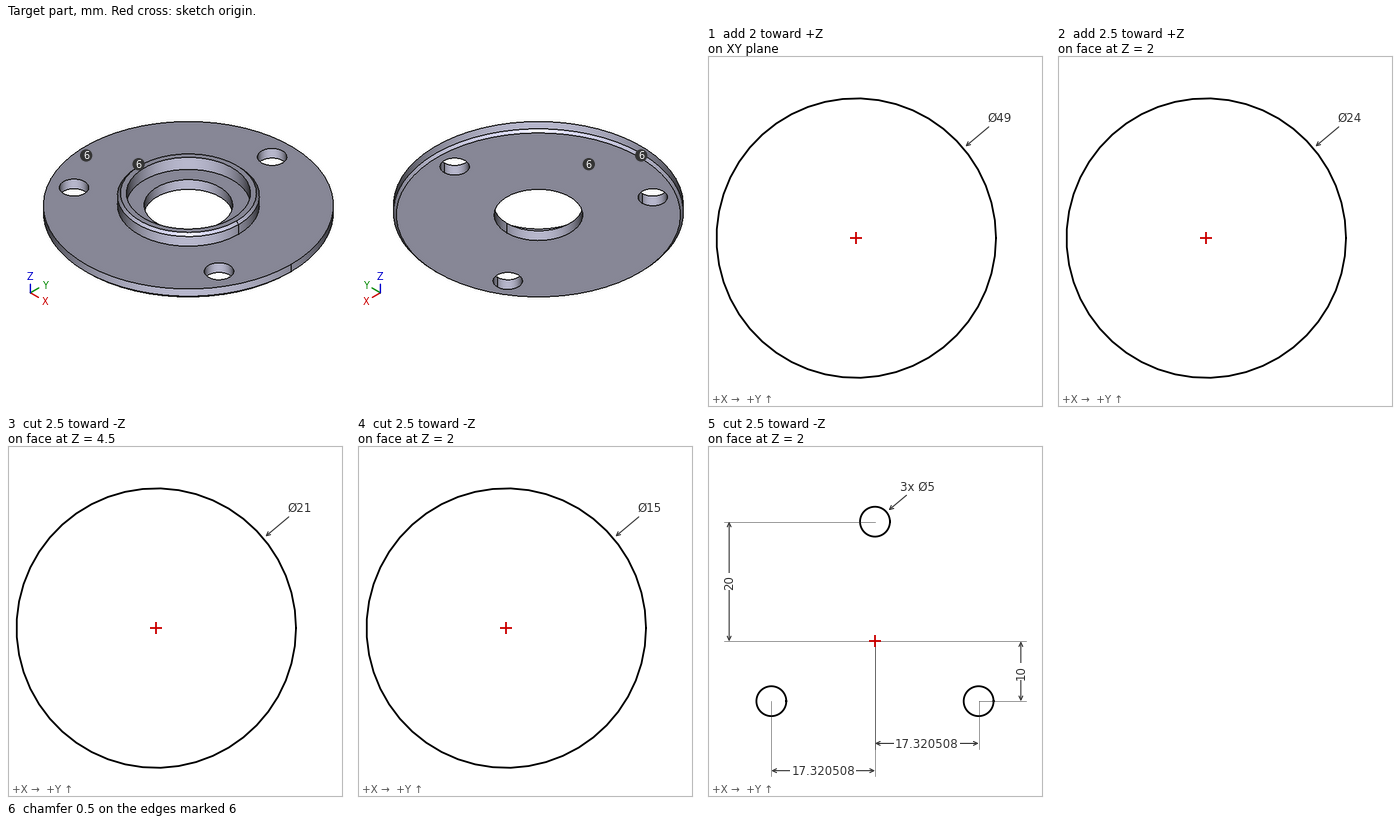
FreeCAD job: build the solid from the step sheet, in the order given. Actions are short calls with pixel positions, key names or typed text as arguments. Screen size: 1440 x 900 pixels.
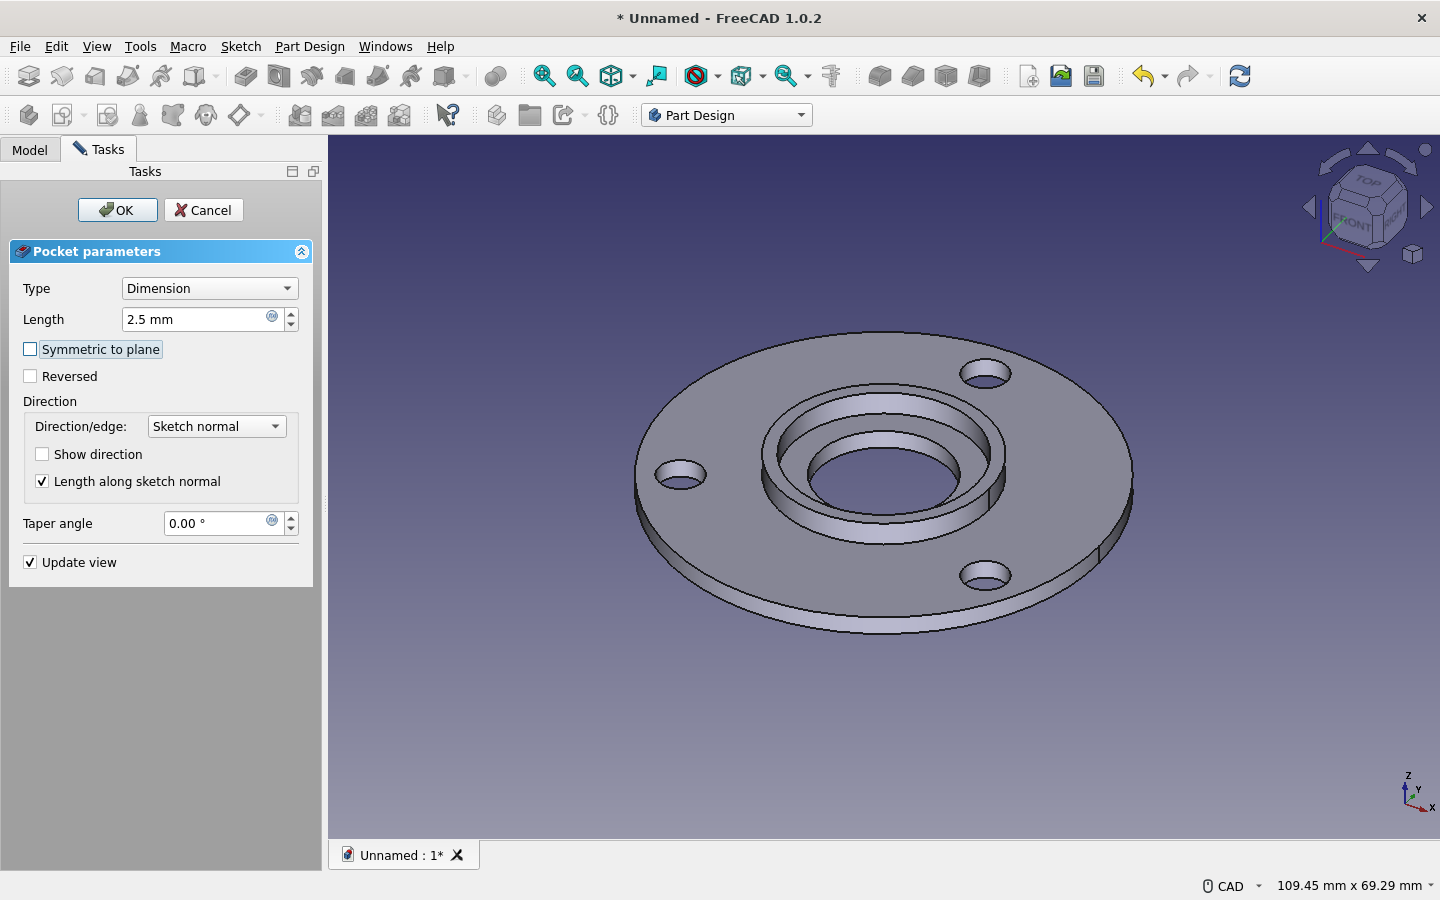
click(118, 210)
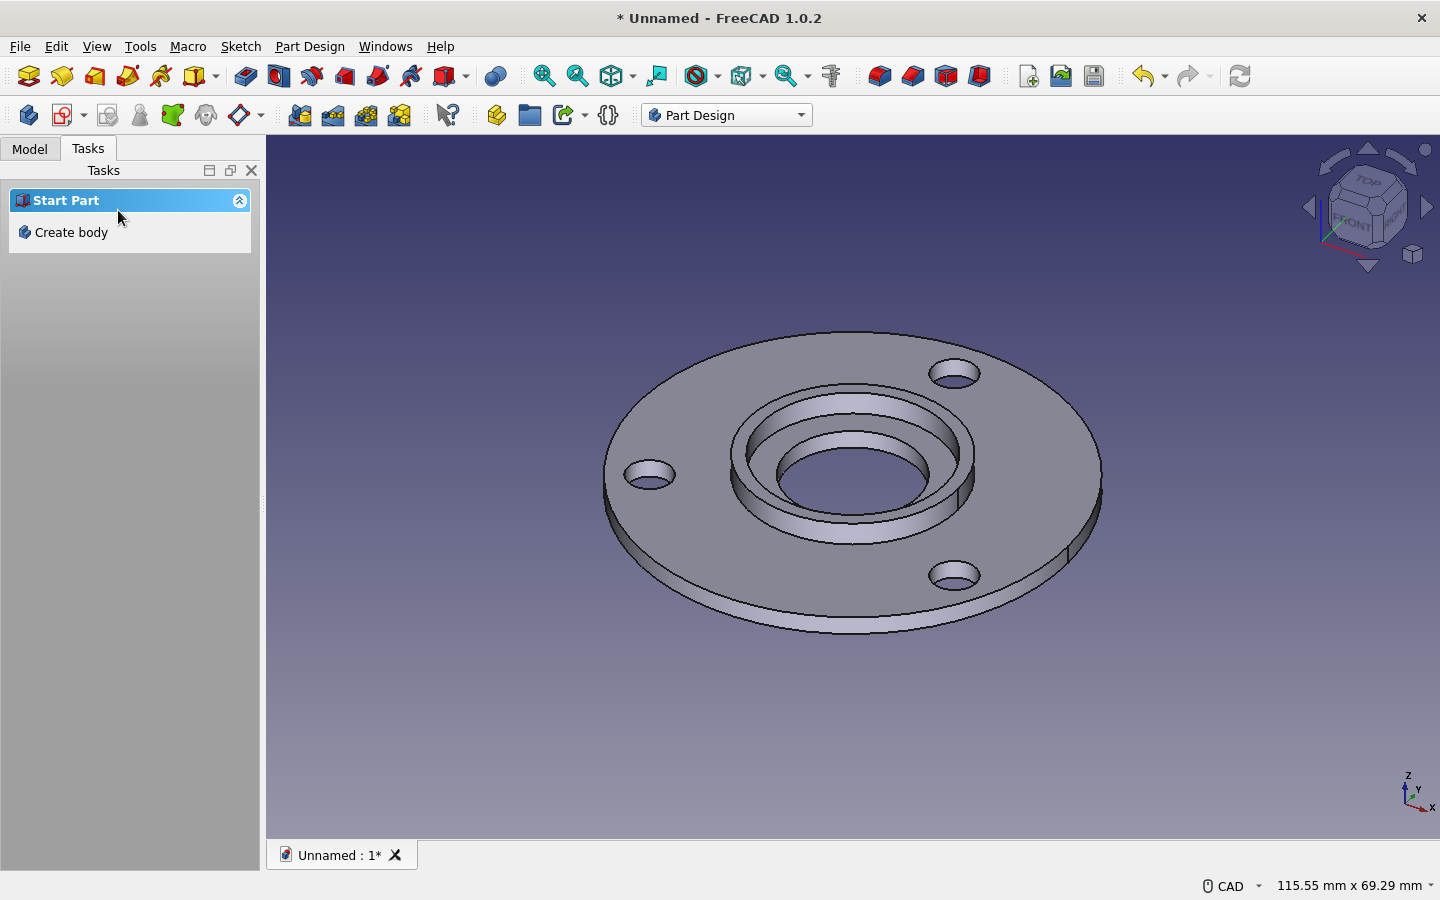
click(732, 460)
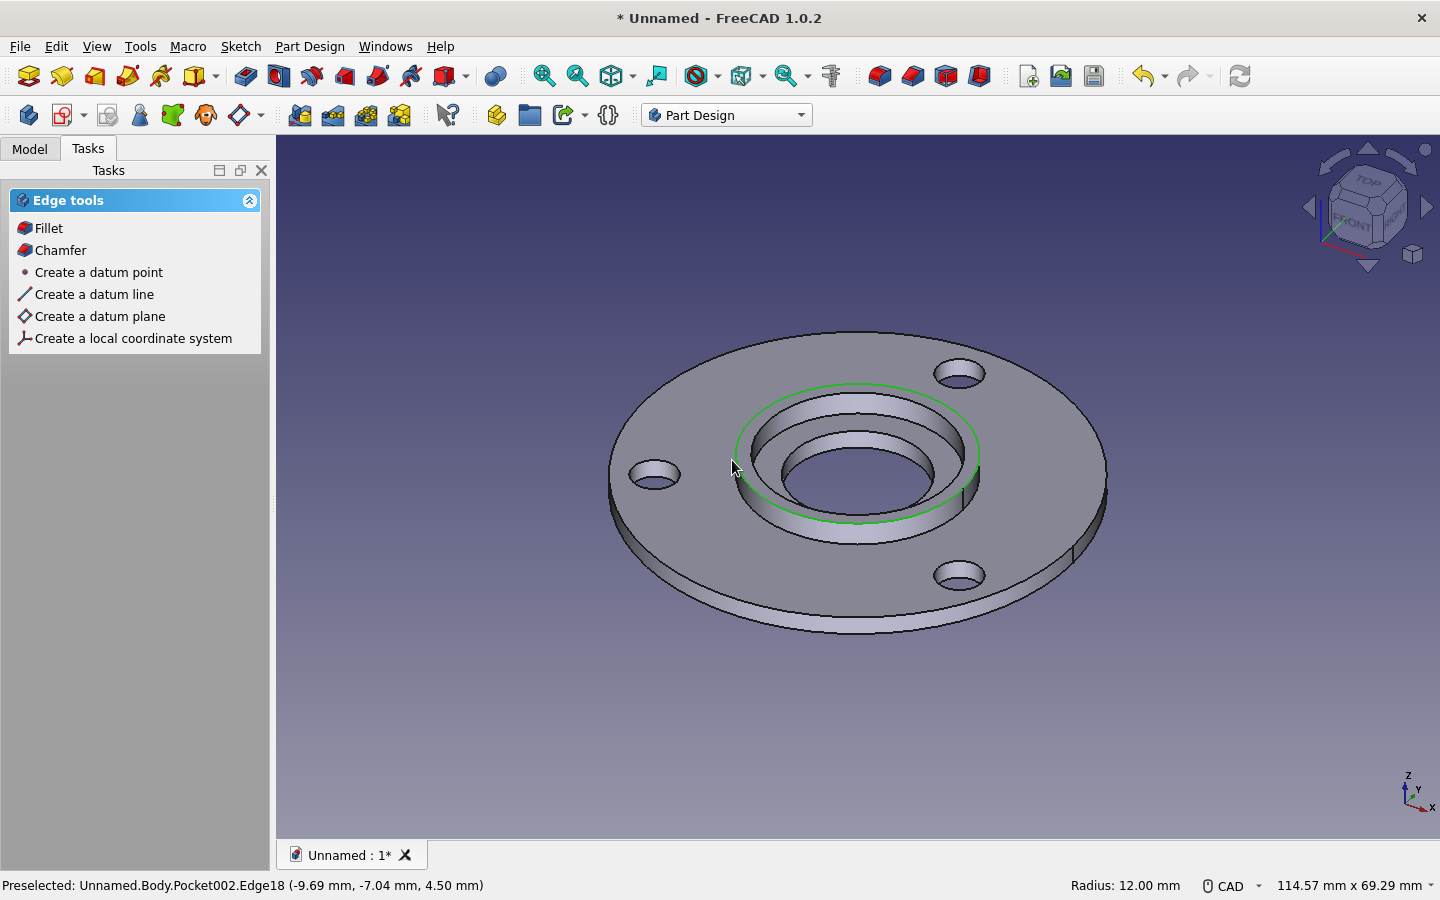
key(0)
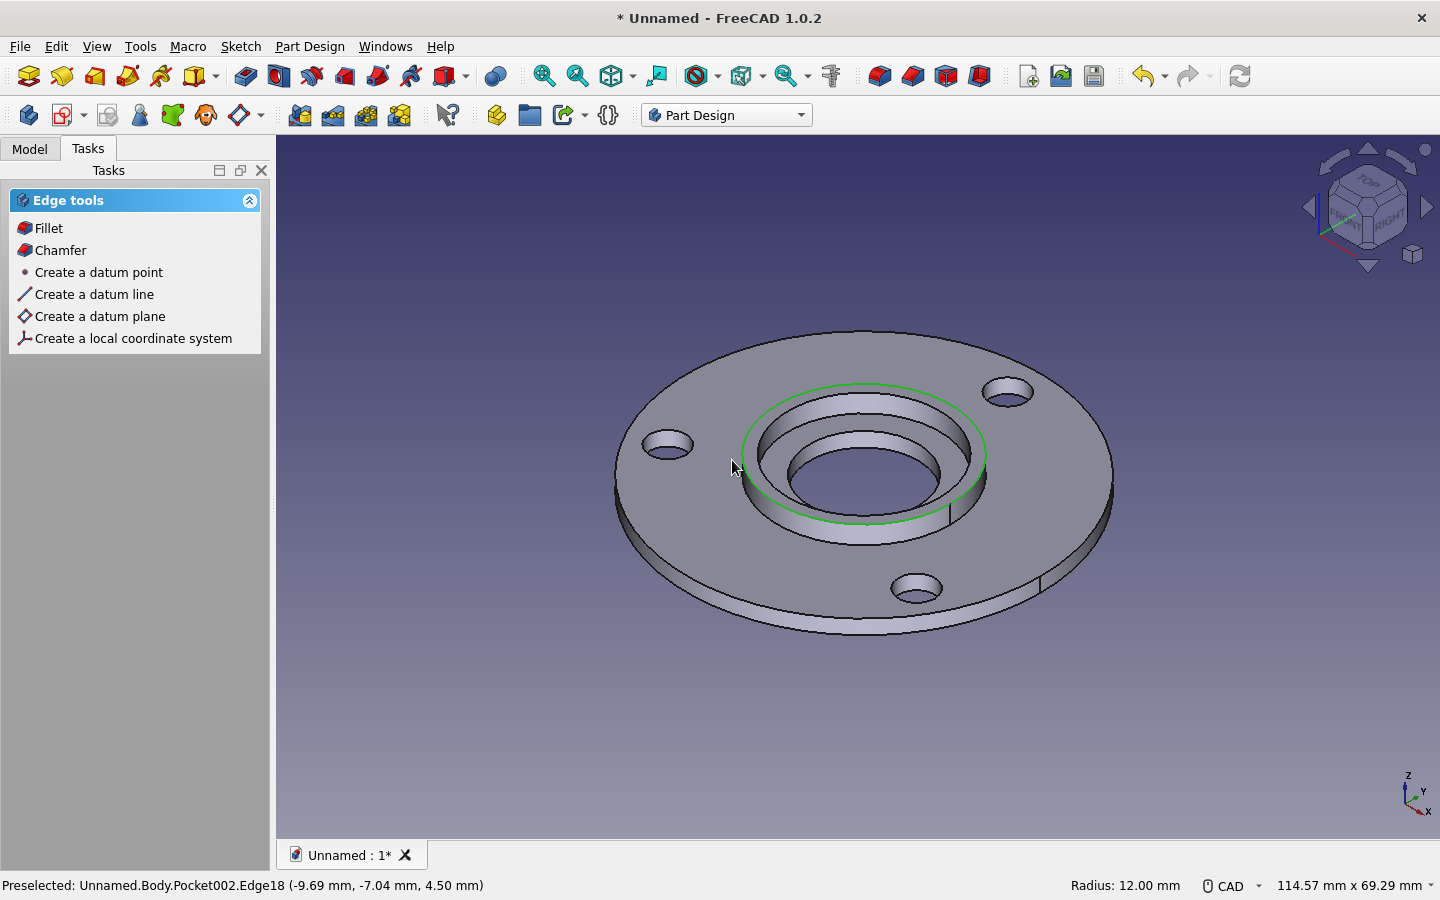
key(2)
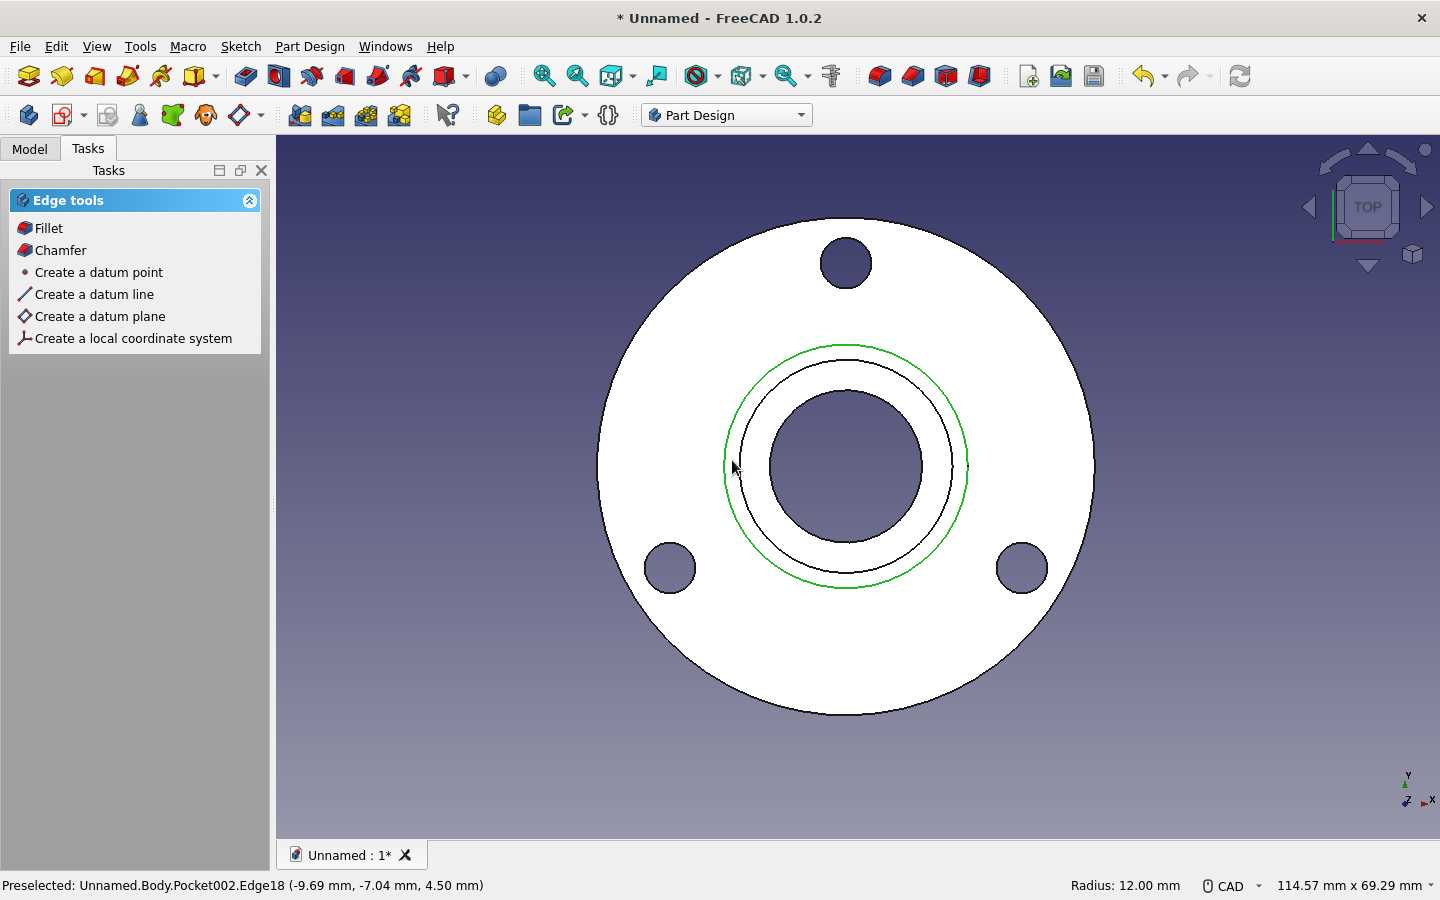
key(1)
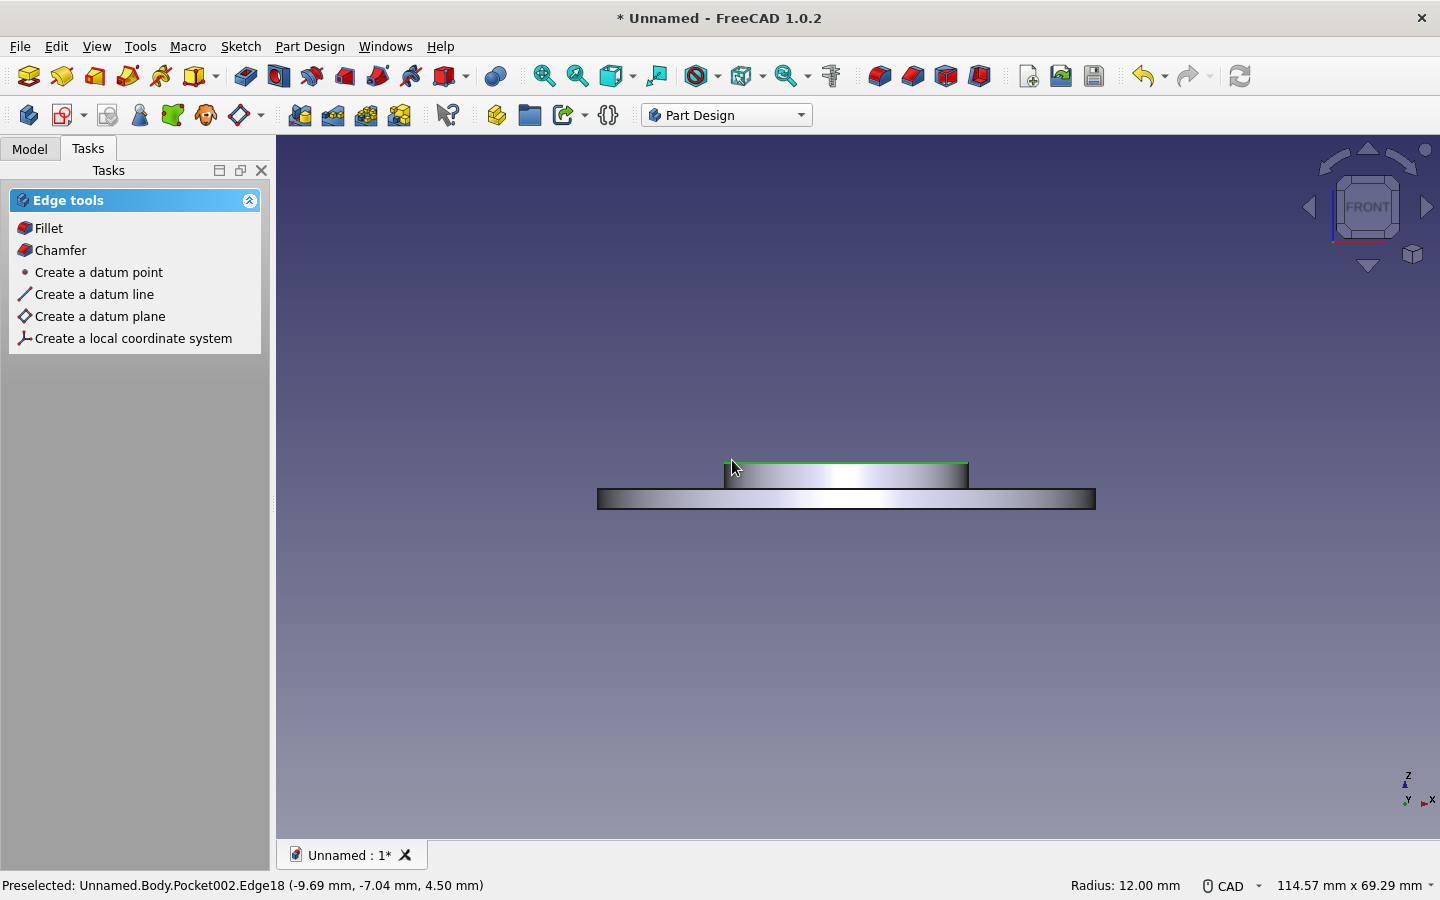
click(545, 76)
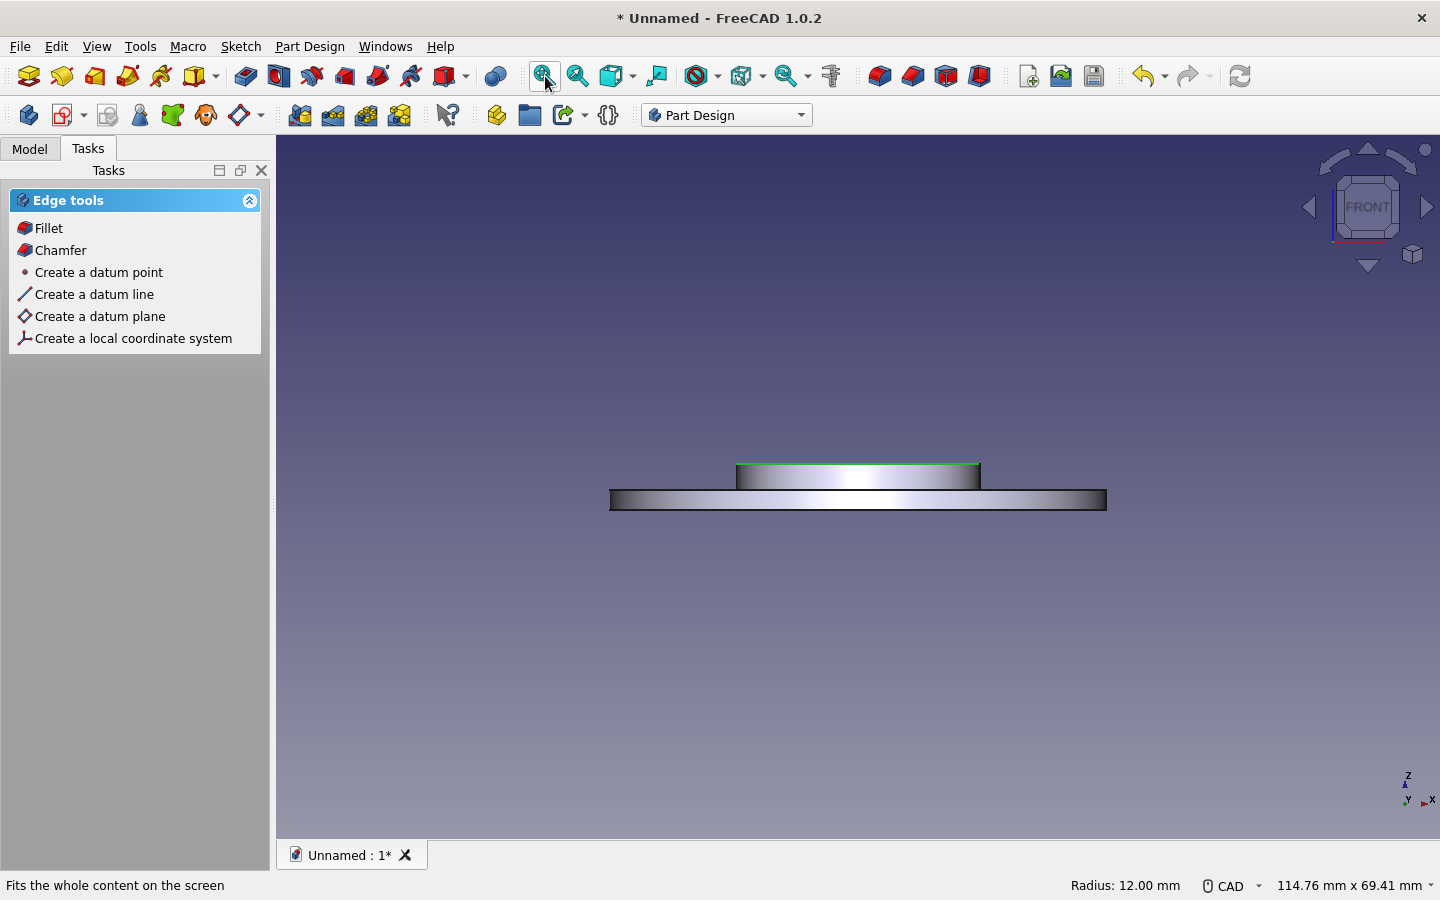
click(657, 509, ctrl)